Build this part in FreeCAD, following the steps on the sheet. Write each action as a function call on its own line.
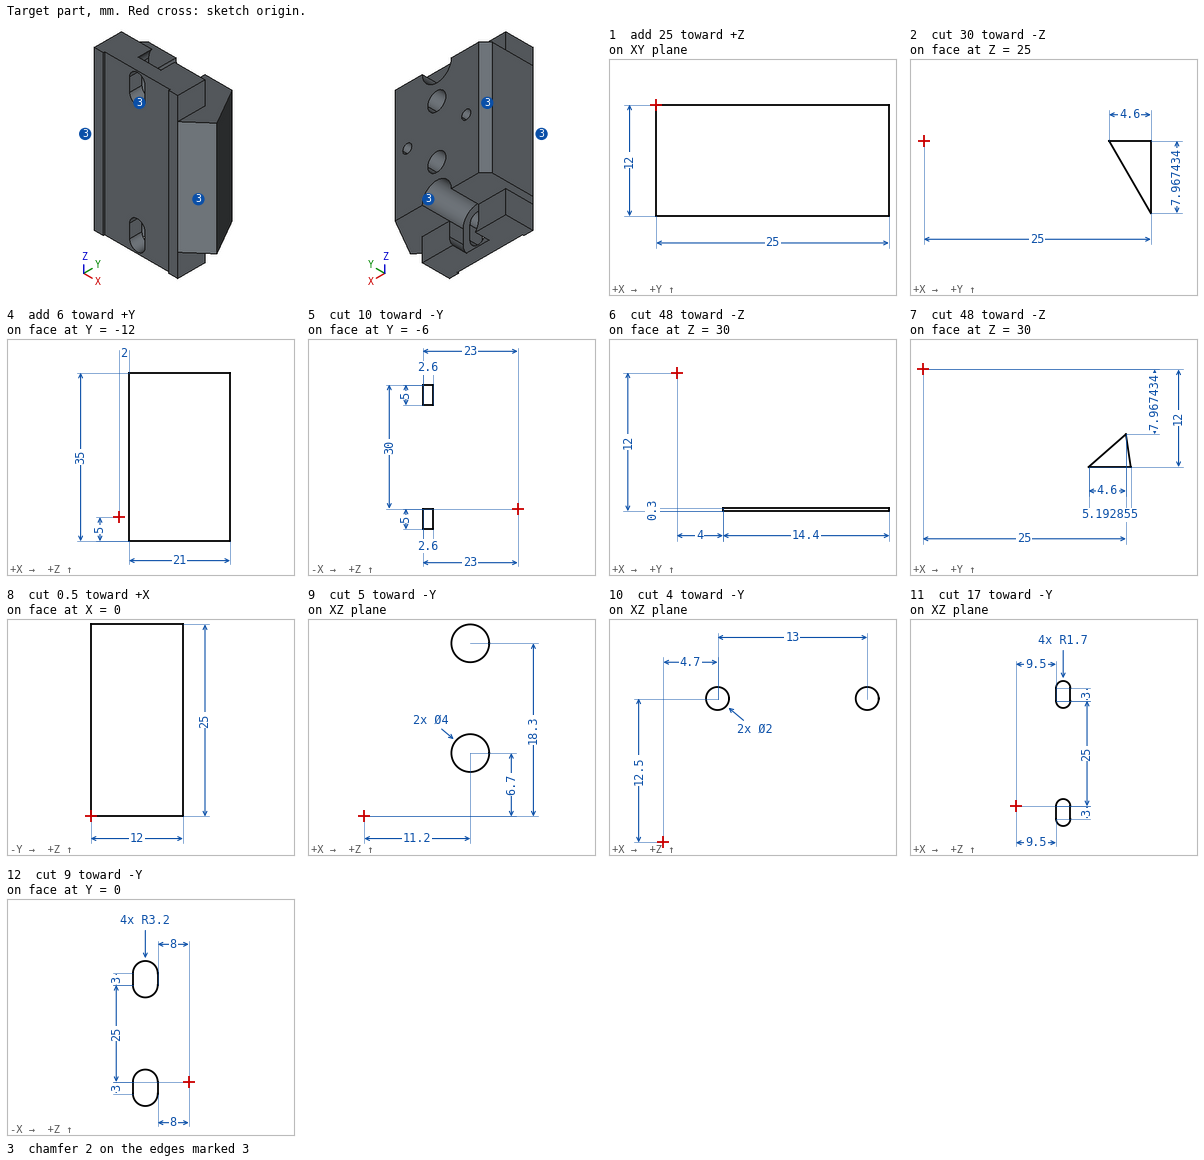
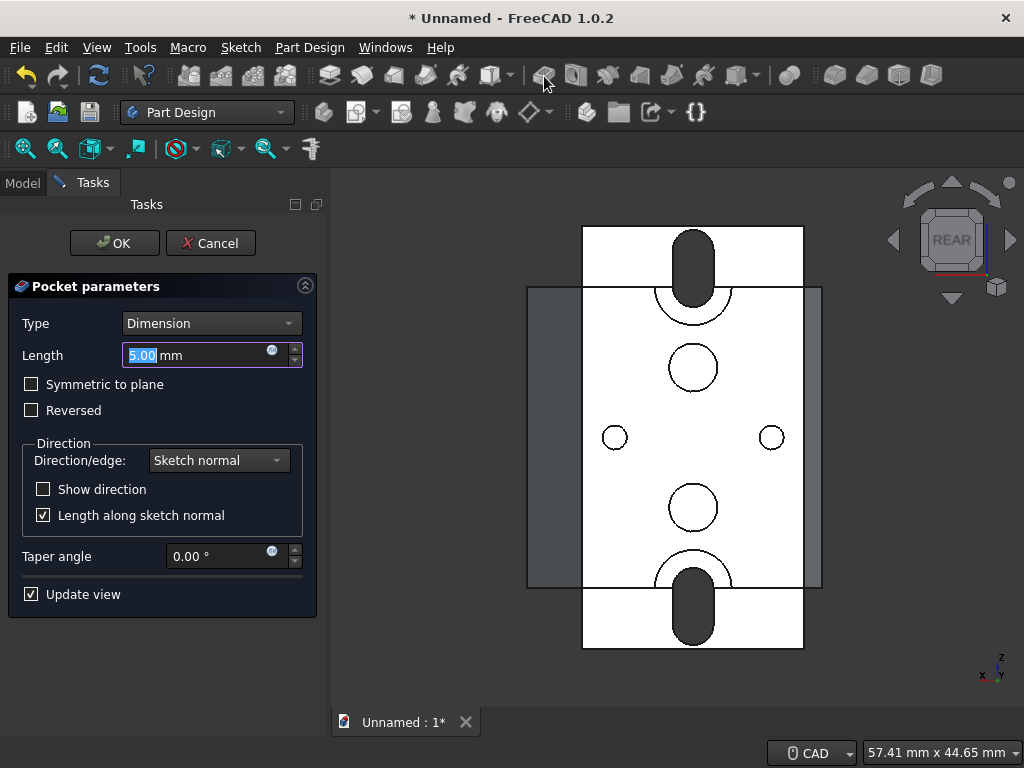
text(9)
key(Tab)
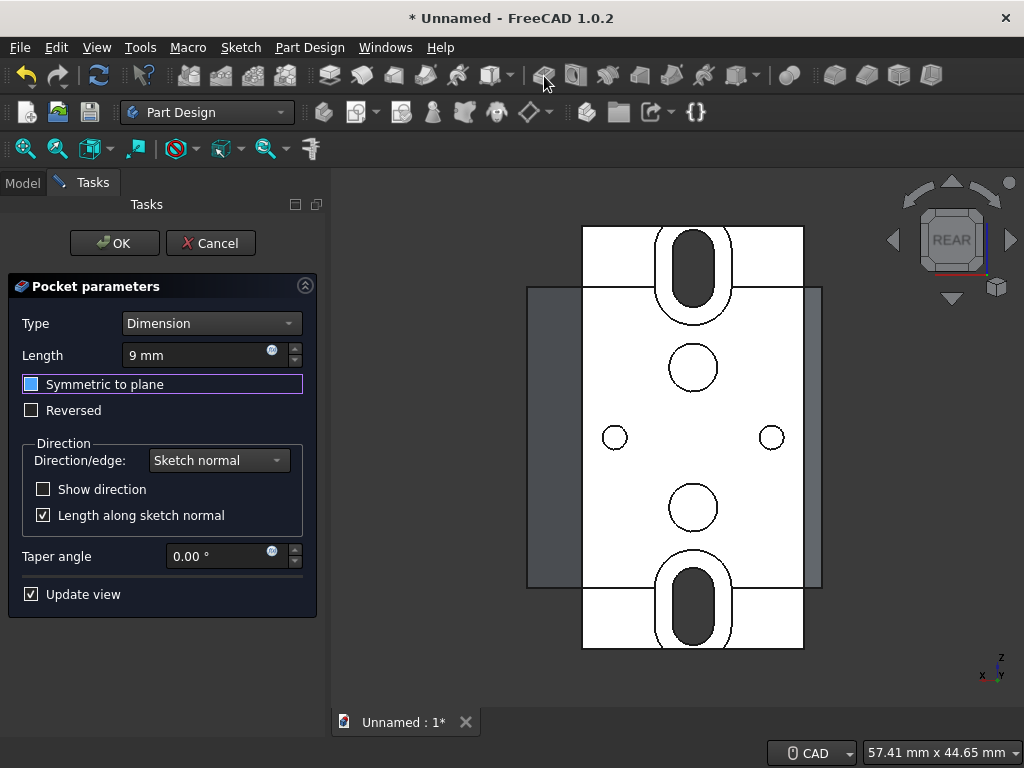
click(115, 243)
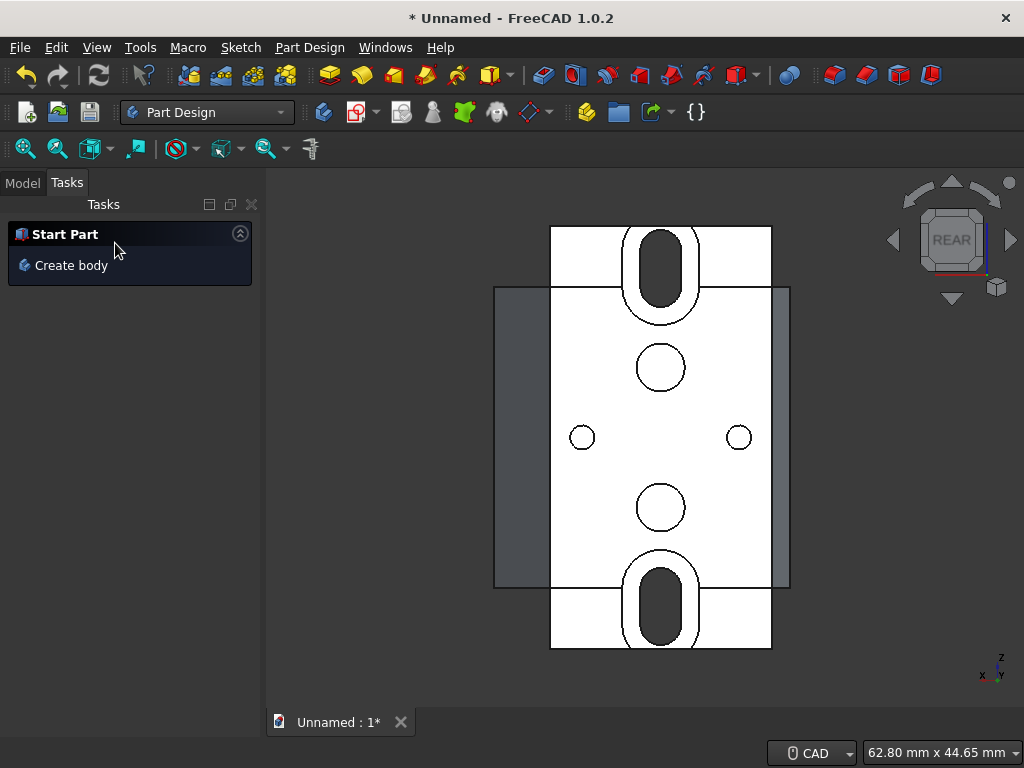
key(0)